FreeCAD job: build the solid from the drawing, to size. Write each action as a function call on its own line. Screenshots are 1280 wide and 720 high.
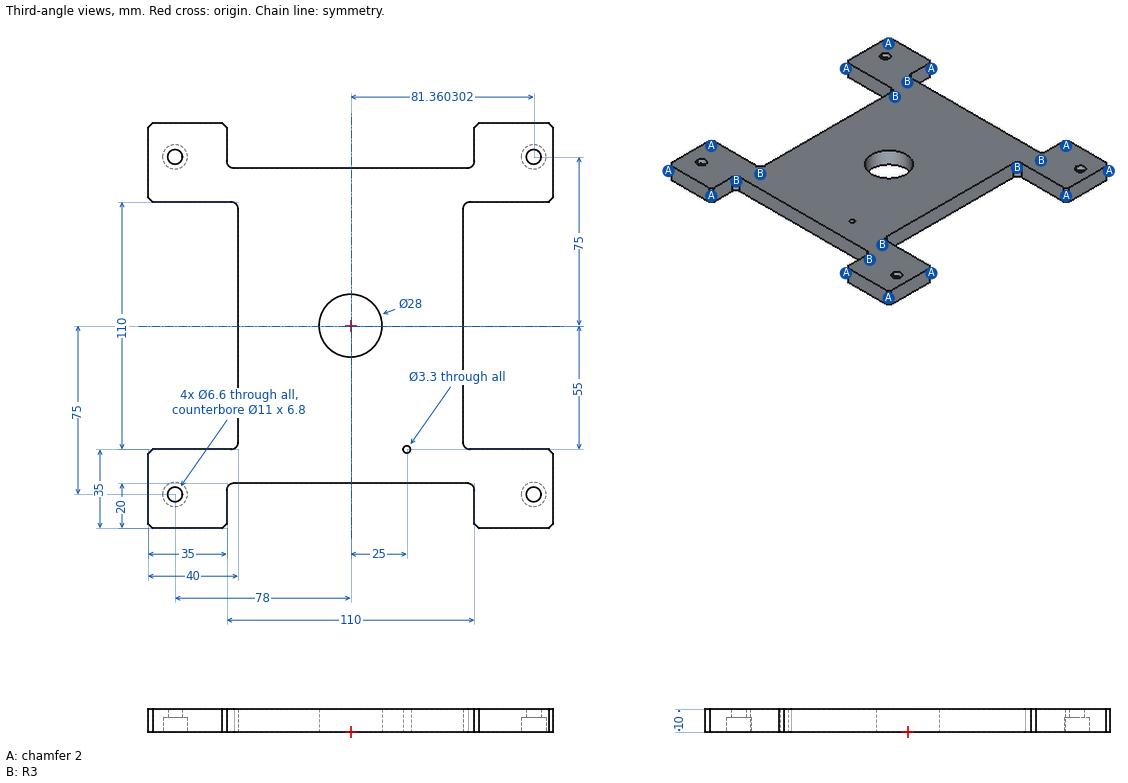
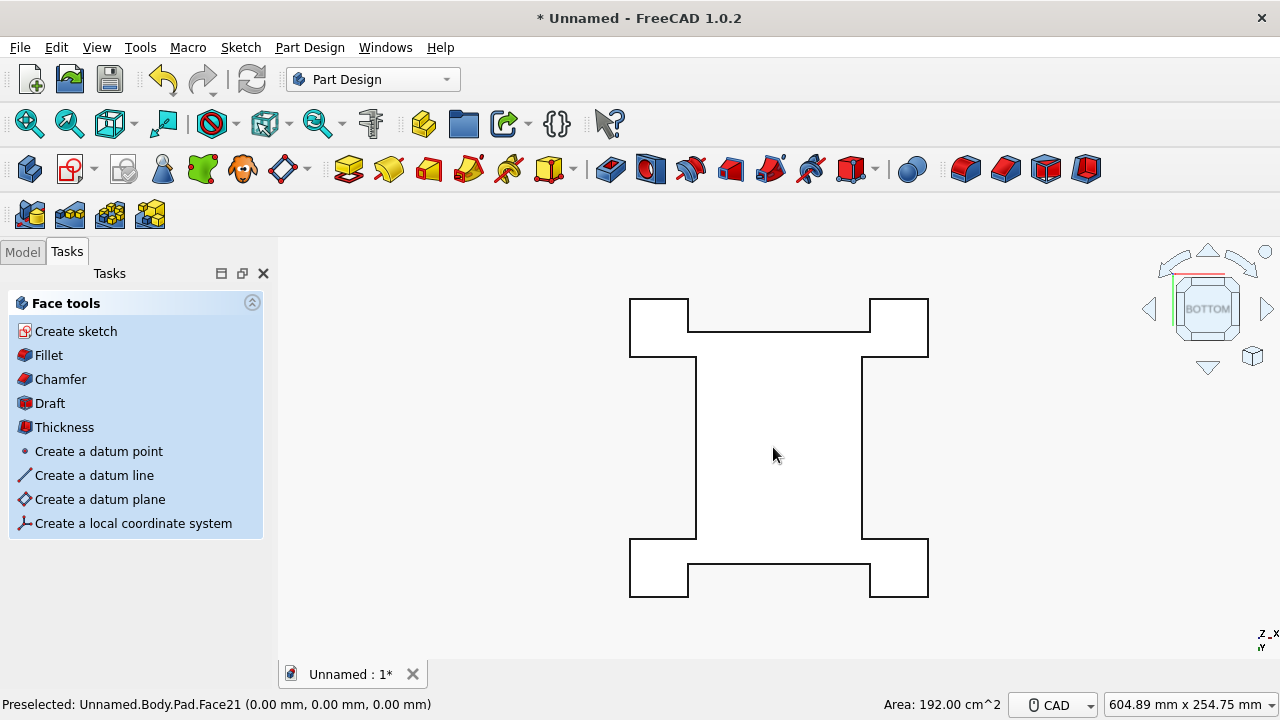
click(70, 170)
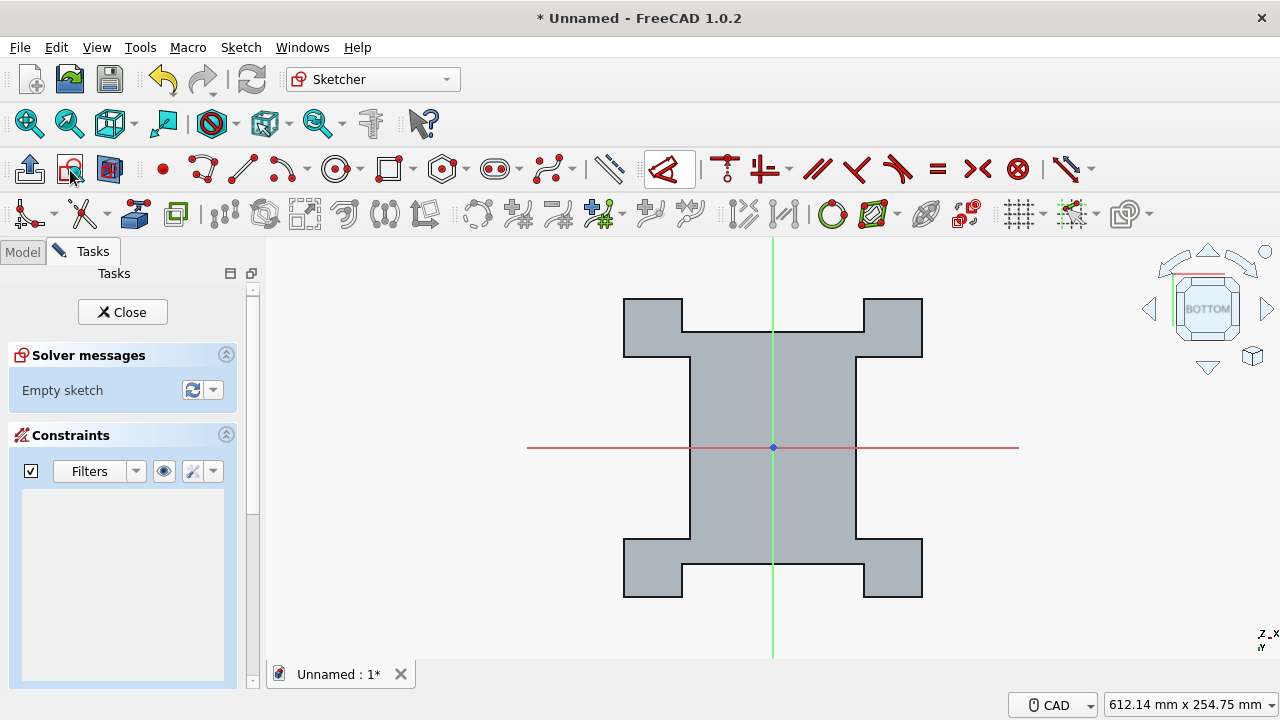
scroll(787, 448, up, 9)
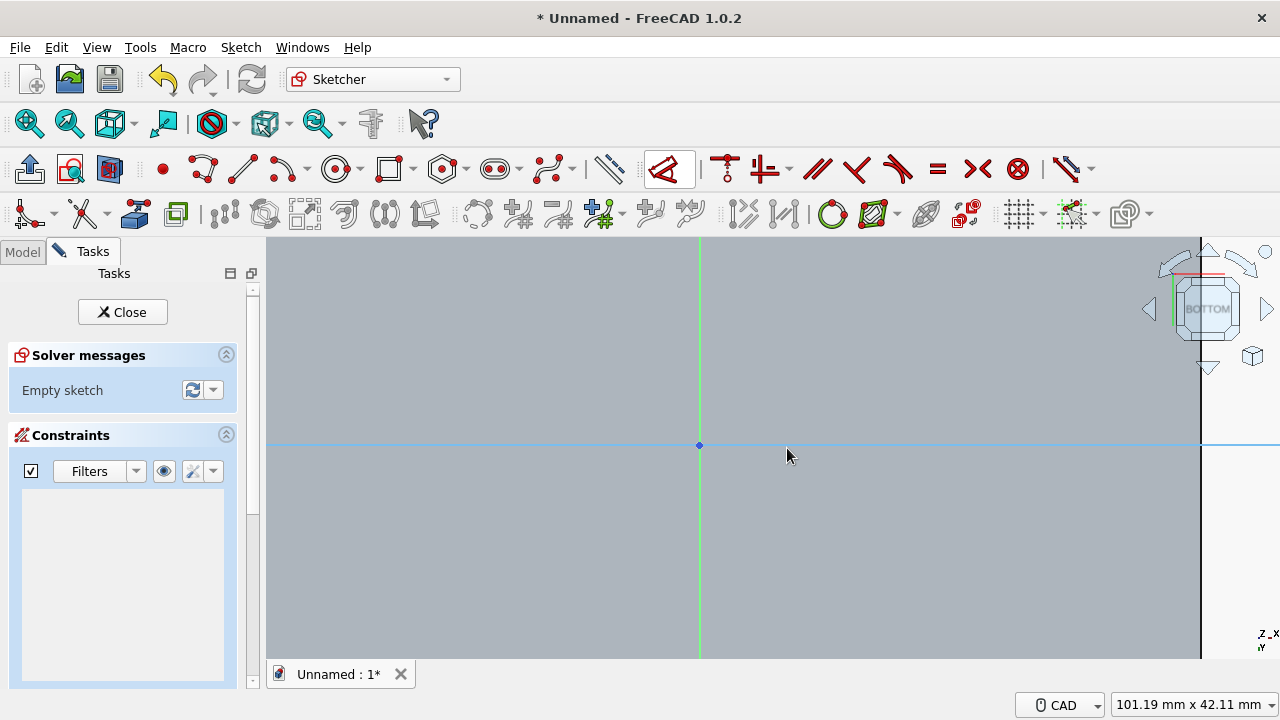
click(336, 170)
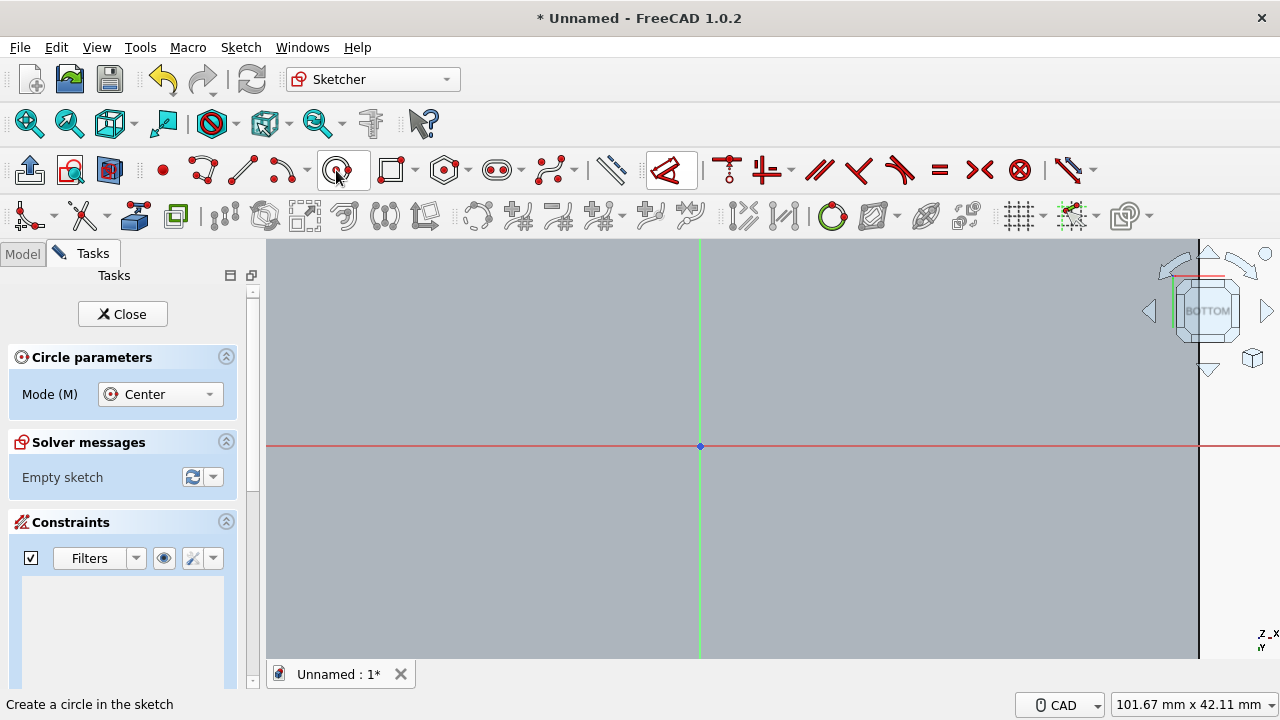
click(700, 446)
click(799, 348)
key(Escape)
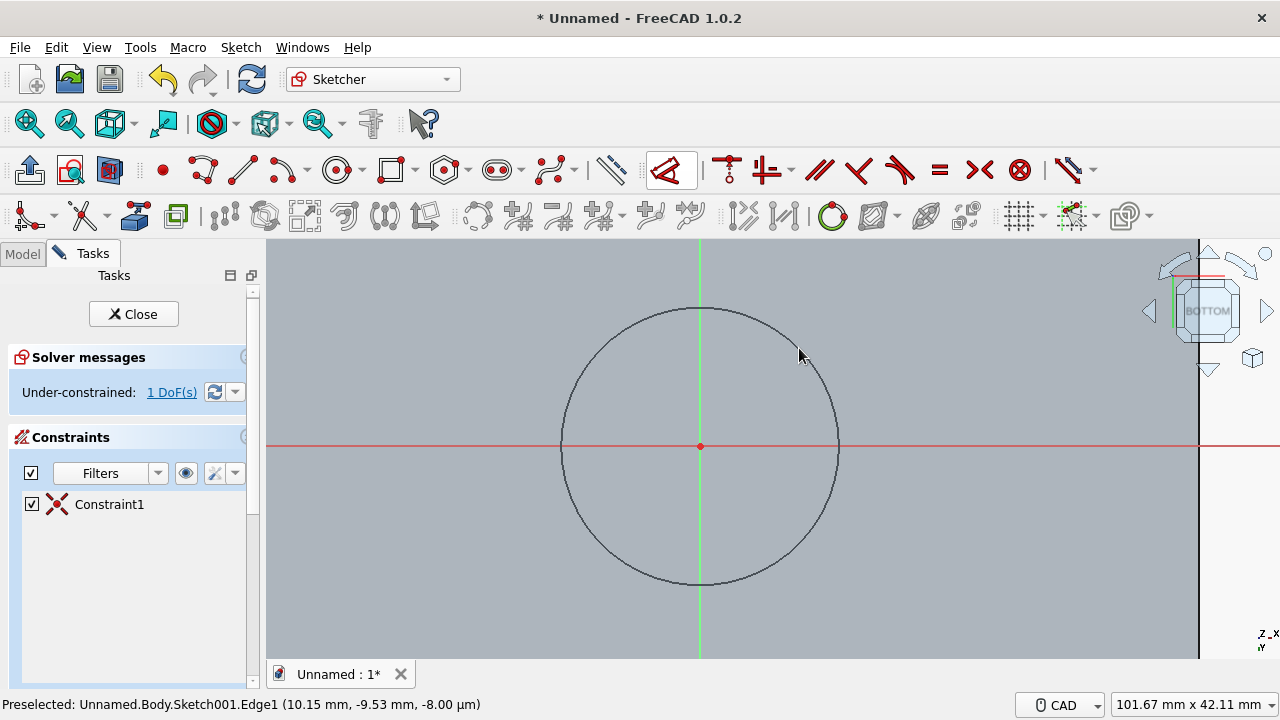
click(798, 348)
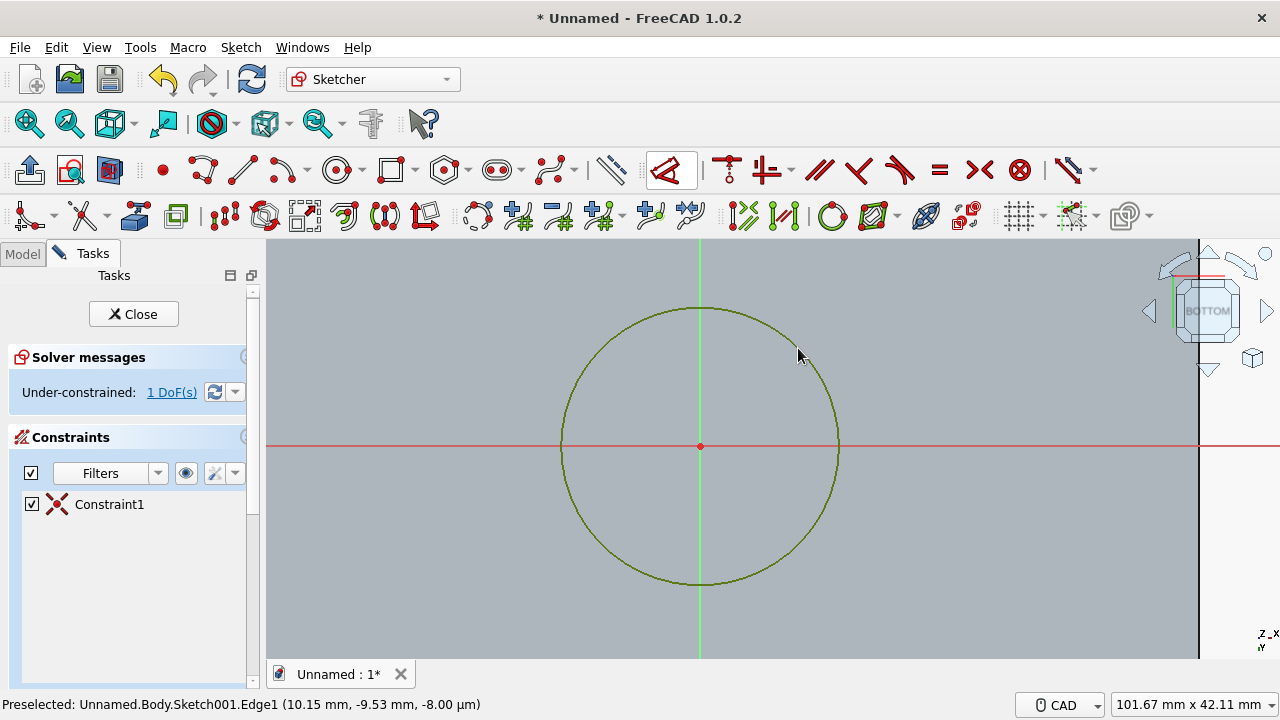
click(692, 170)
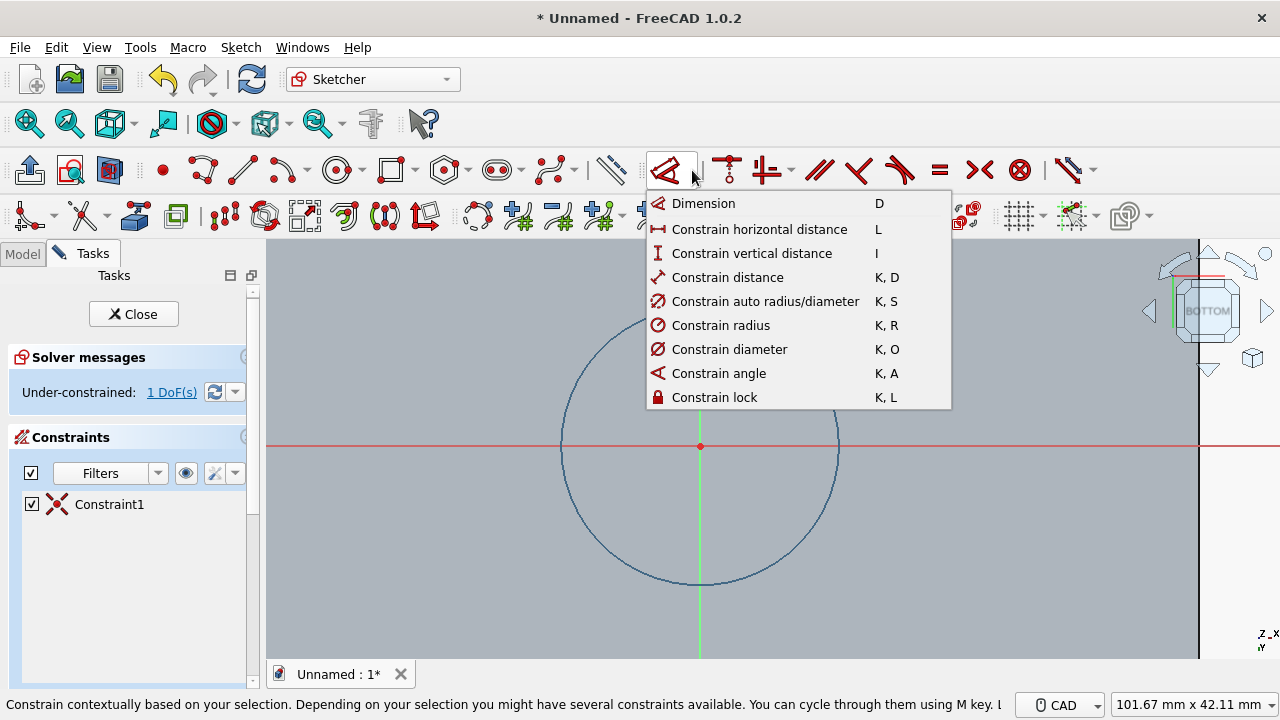
click(799, 349)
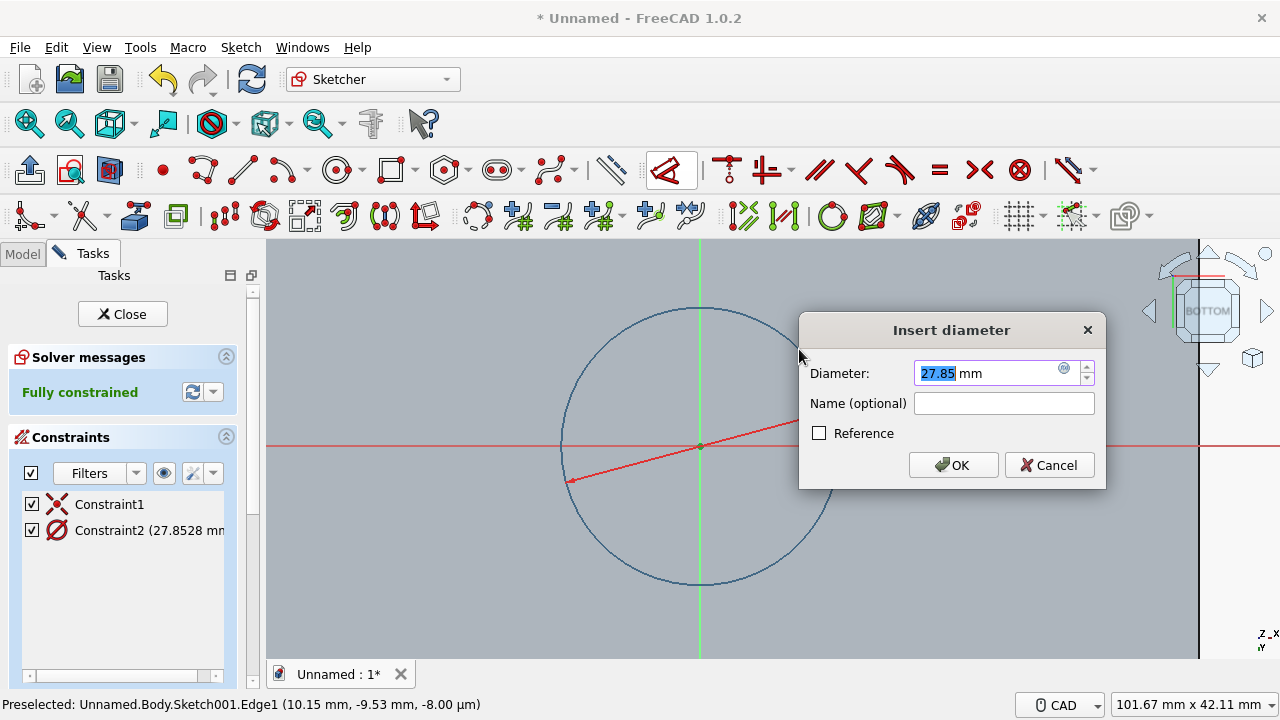
text(28)
key(Return)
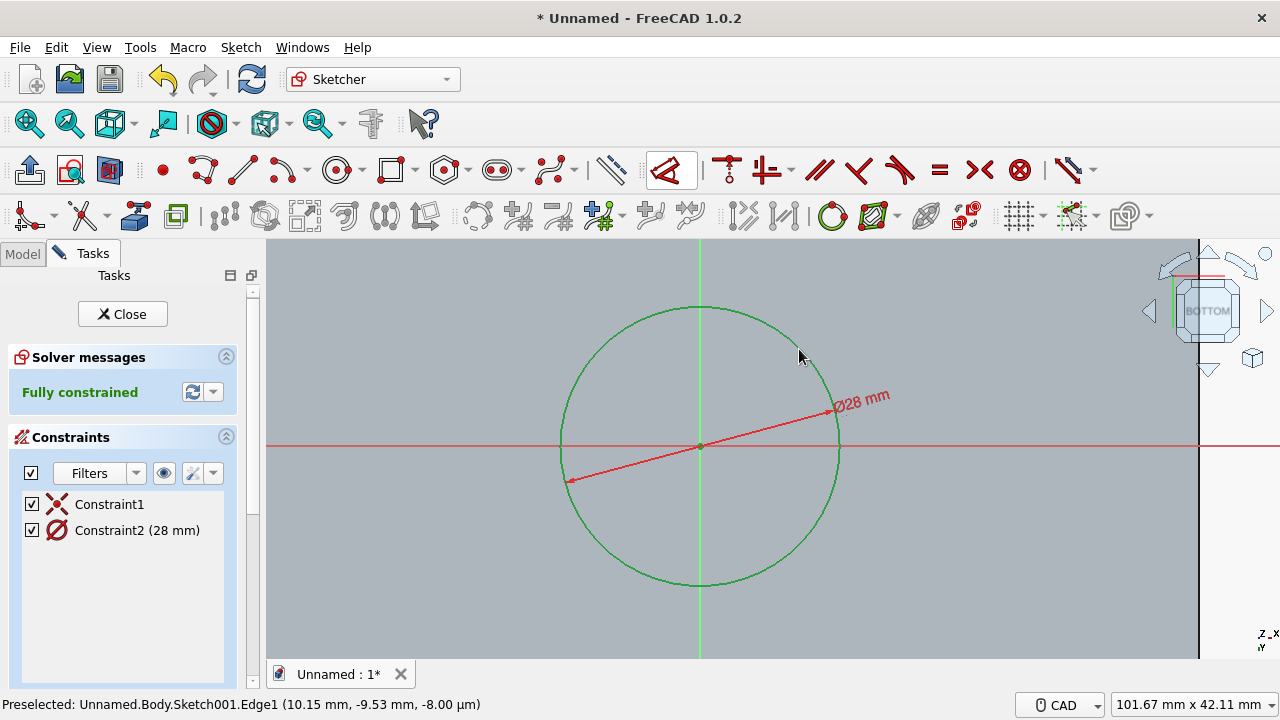
click(123, 314)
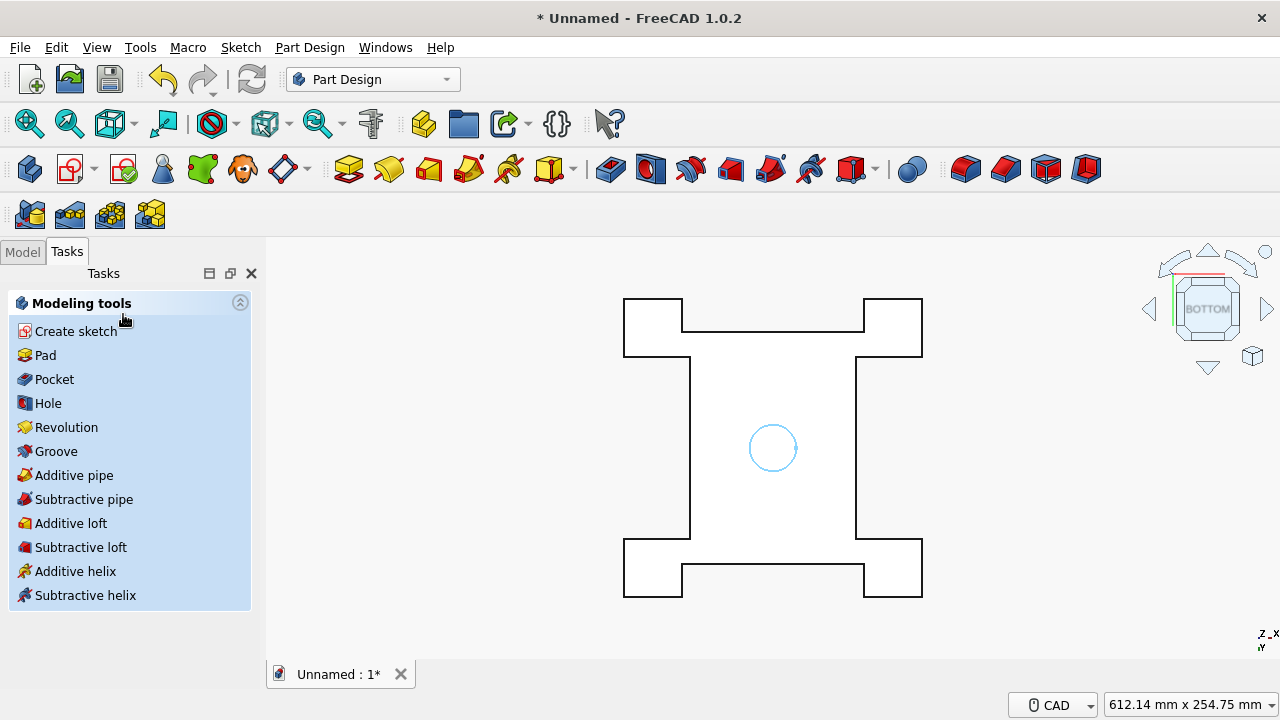
click(612, 170)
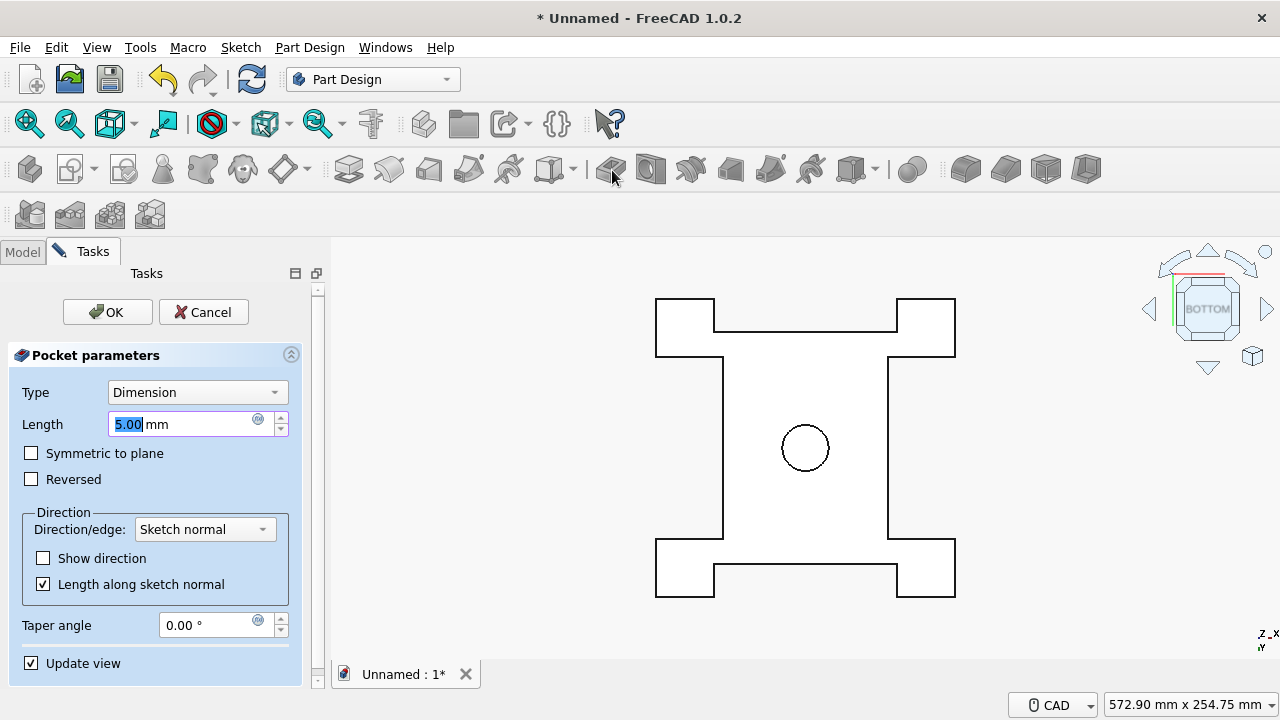
click(198, 392)